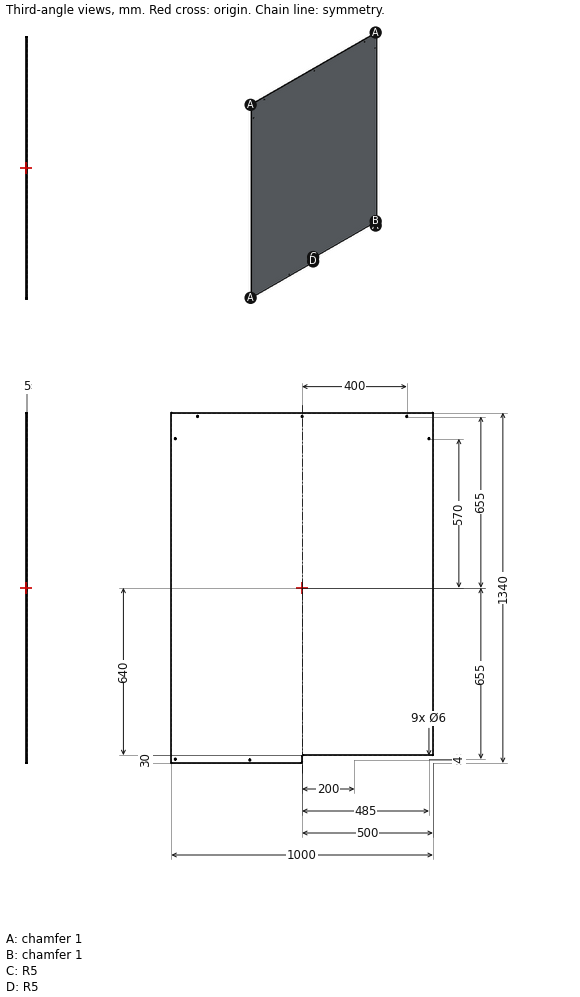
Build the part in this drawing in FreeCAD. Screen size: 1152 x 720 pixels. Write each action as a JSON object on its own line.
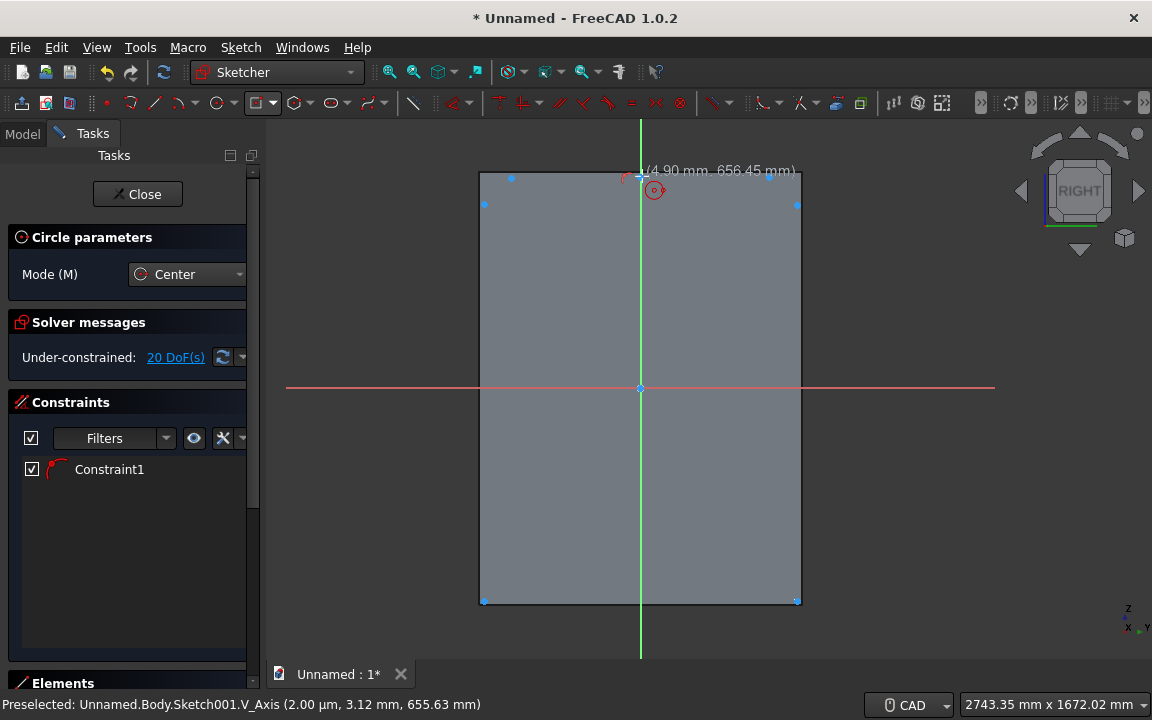
{"action": "scroll", "coordinate": [705, 601], "scroll_direction": "up", "scroll_amount": 16}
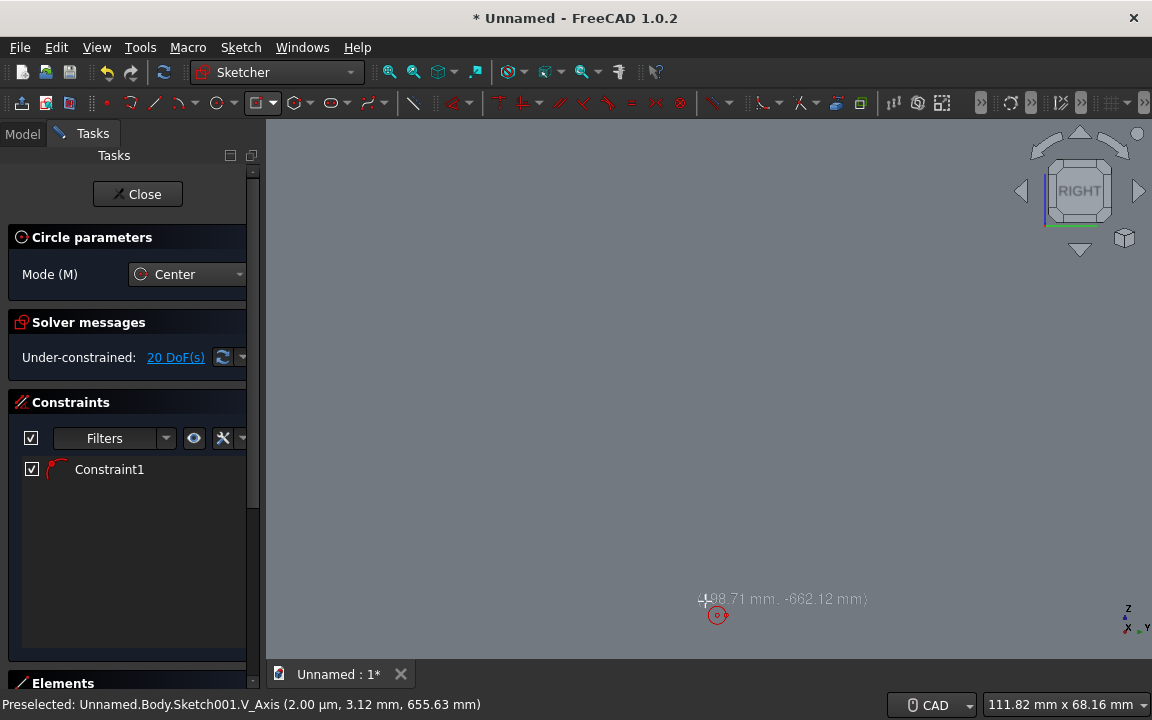
{"action": "scroll", "coordinate": [705, 602], "scroll_direction": "down", "scroll_amount": 16}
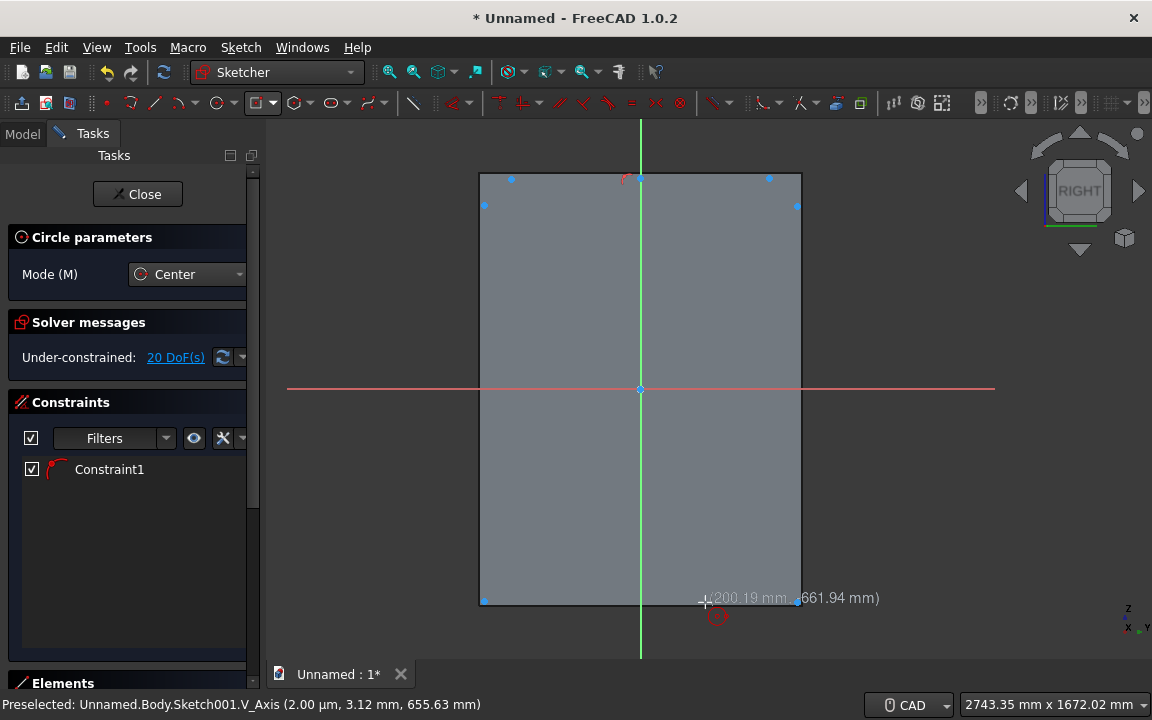
{"action": "left_click", "coordinate": [705, 602]}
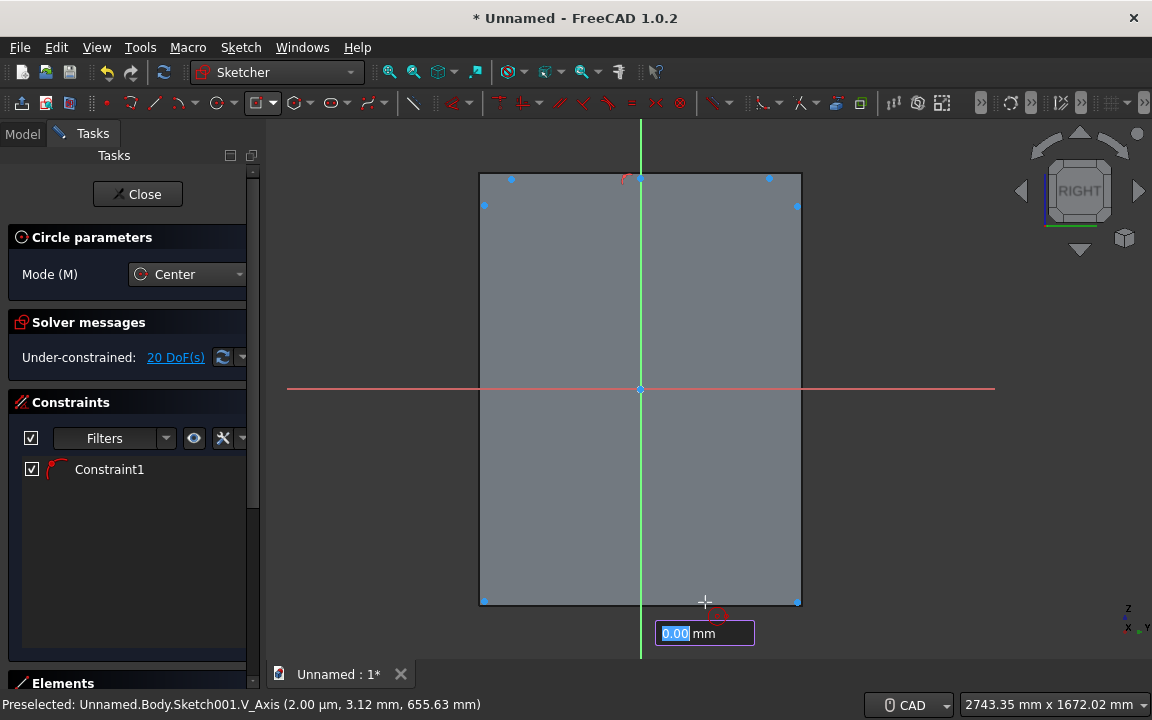
{"action": "scroll", "coordinate": [706, 601], "scroll_direction": "up", "scroll_amount": 14}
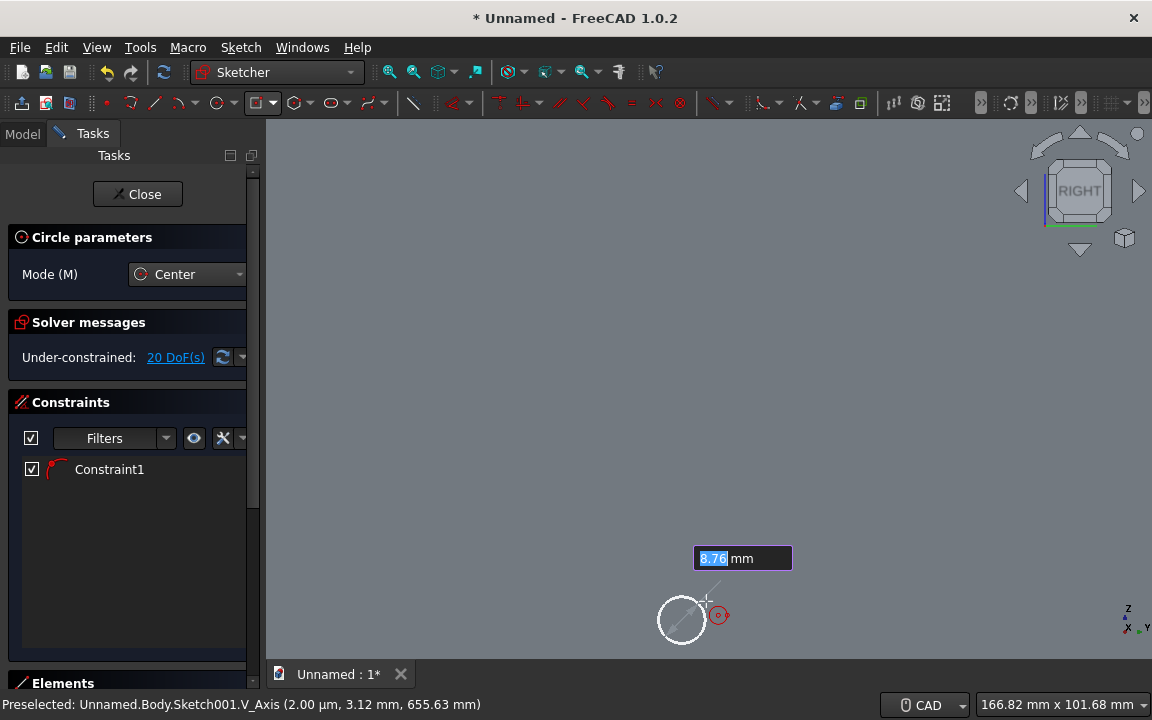
{"action": "left_click", "coordinate": [700, 592]}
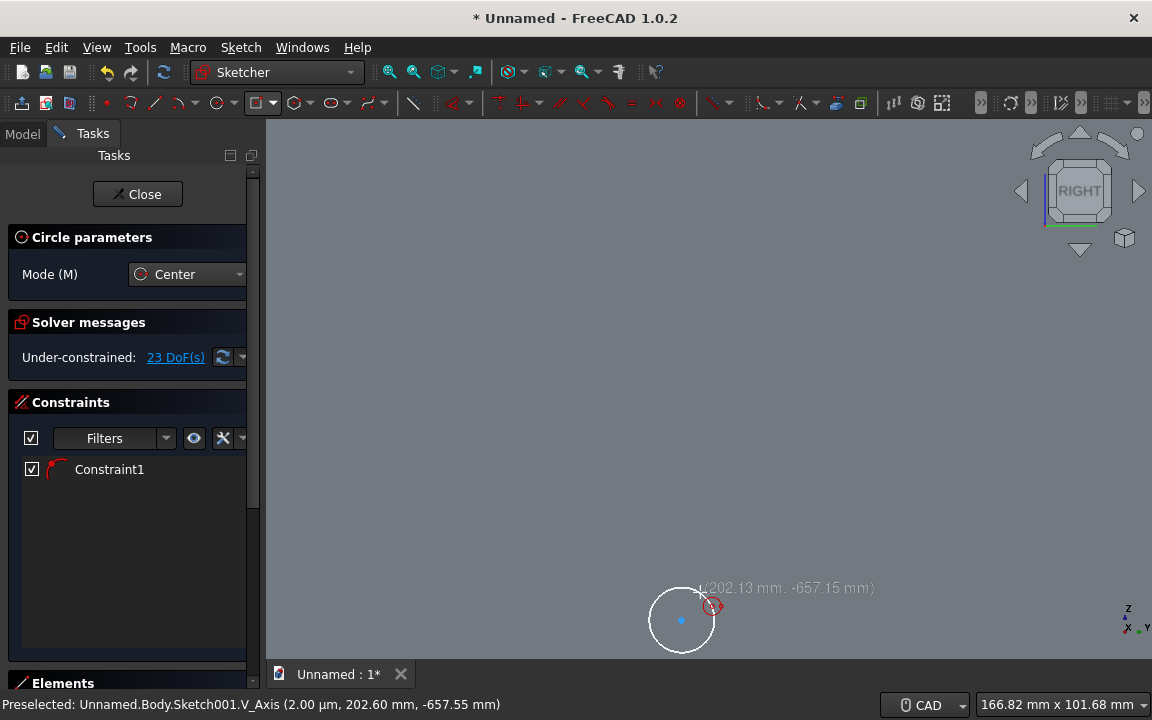
{"action": "scroll", "coordinate": [694, 561], "scroll_direction": "down", "scroll_amount": 15}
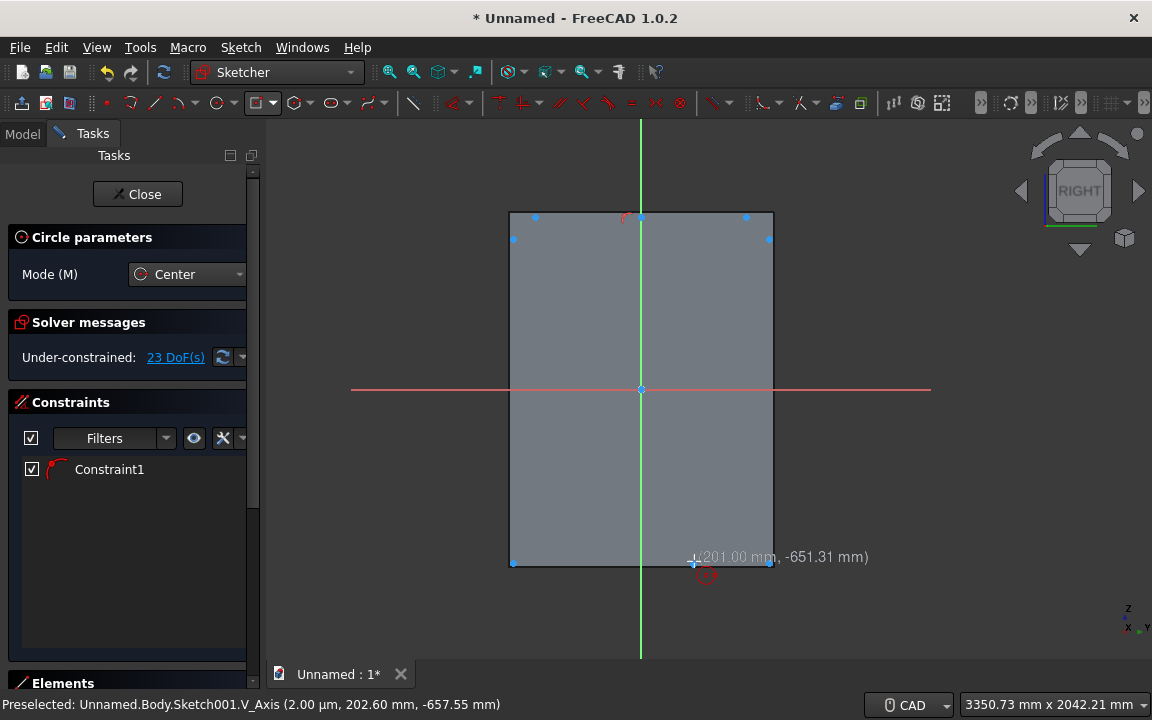
{"action": "scroll", "coordinate": [588, 564], "scroll_direction": "up", "scroll_amount": 17}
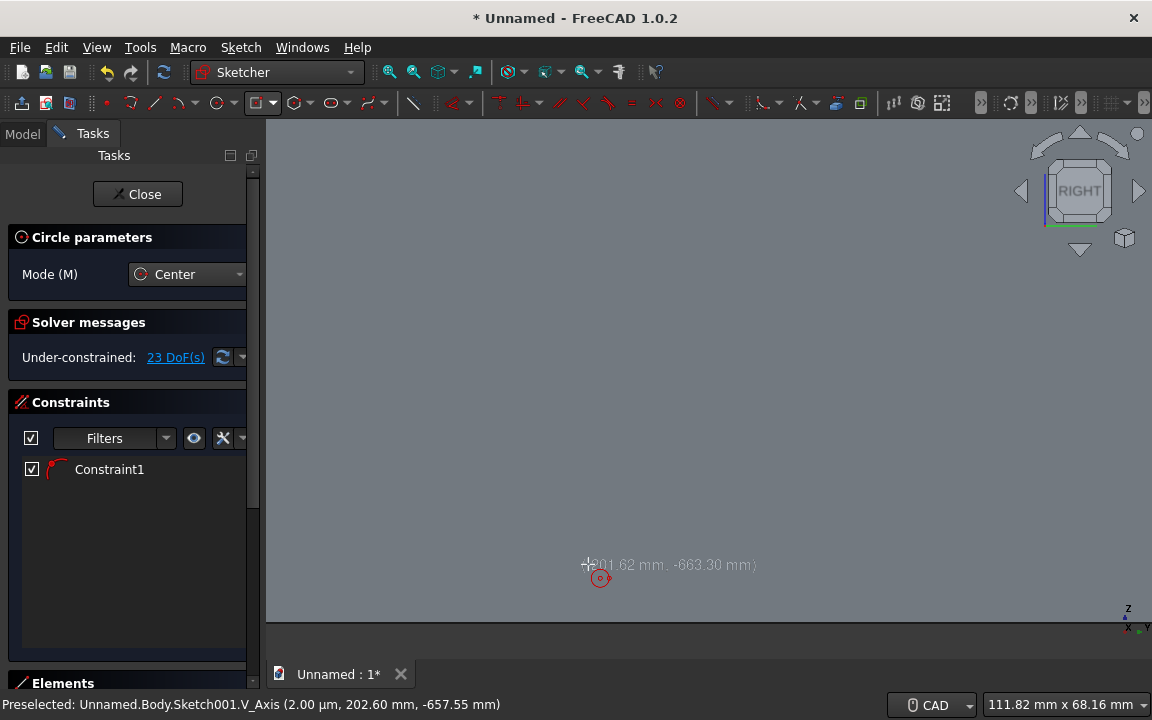
{"action": "scroll", "coordinate": [575, 604], "scroll_direction": "down", "scroll_amount": 16}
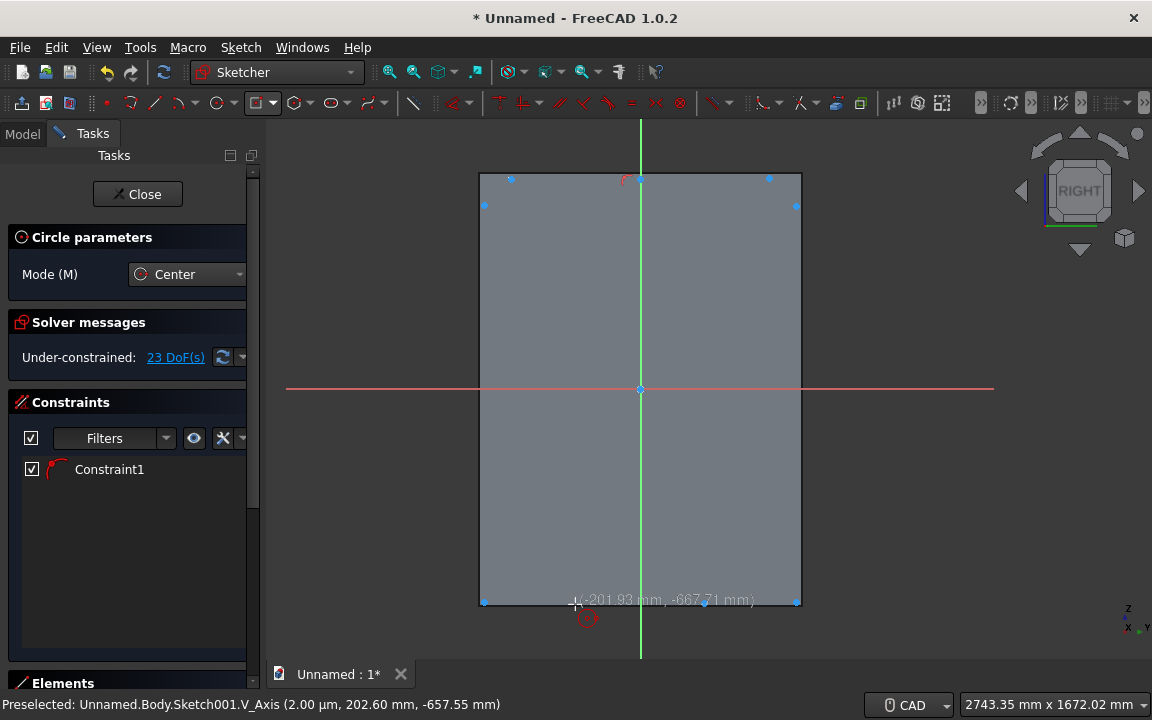
{"action": "left_click", "coordinate": [576, 602]}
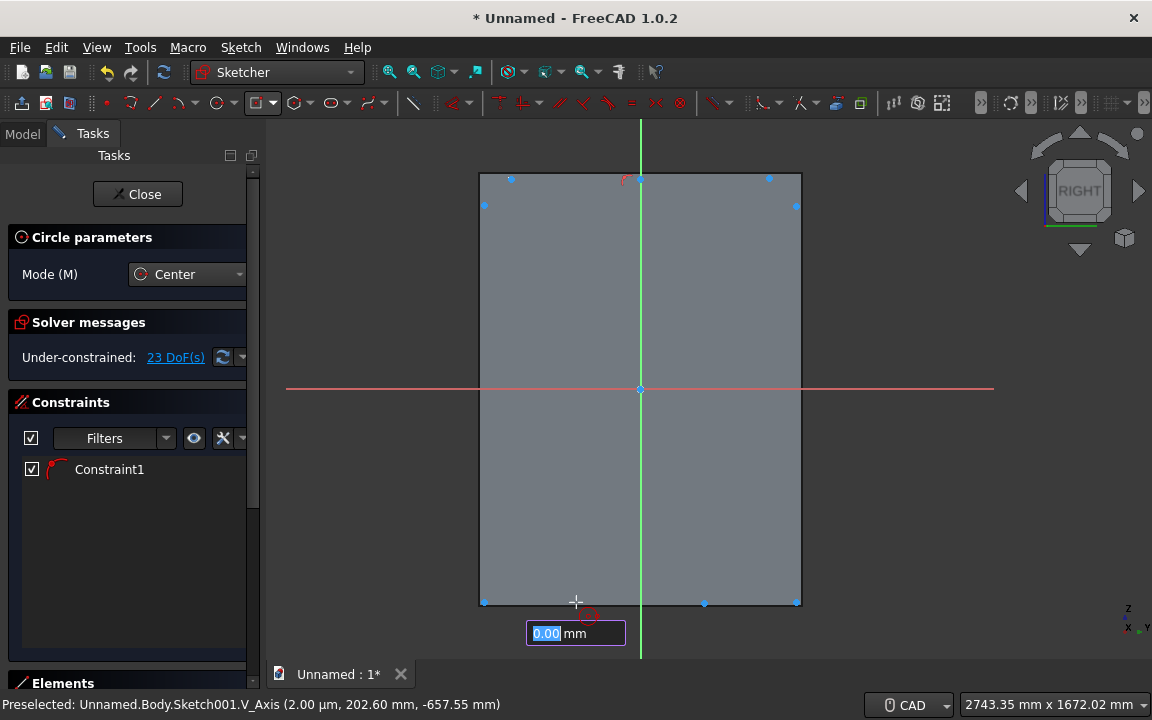
{"action": "scroll", "coordinate": [577, 601], "scroll_direction": "up", "scroll_amount": 14}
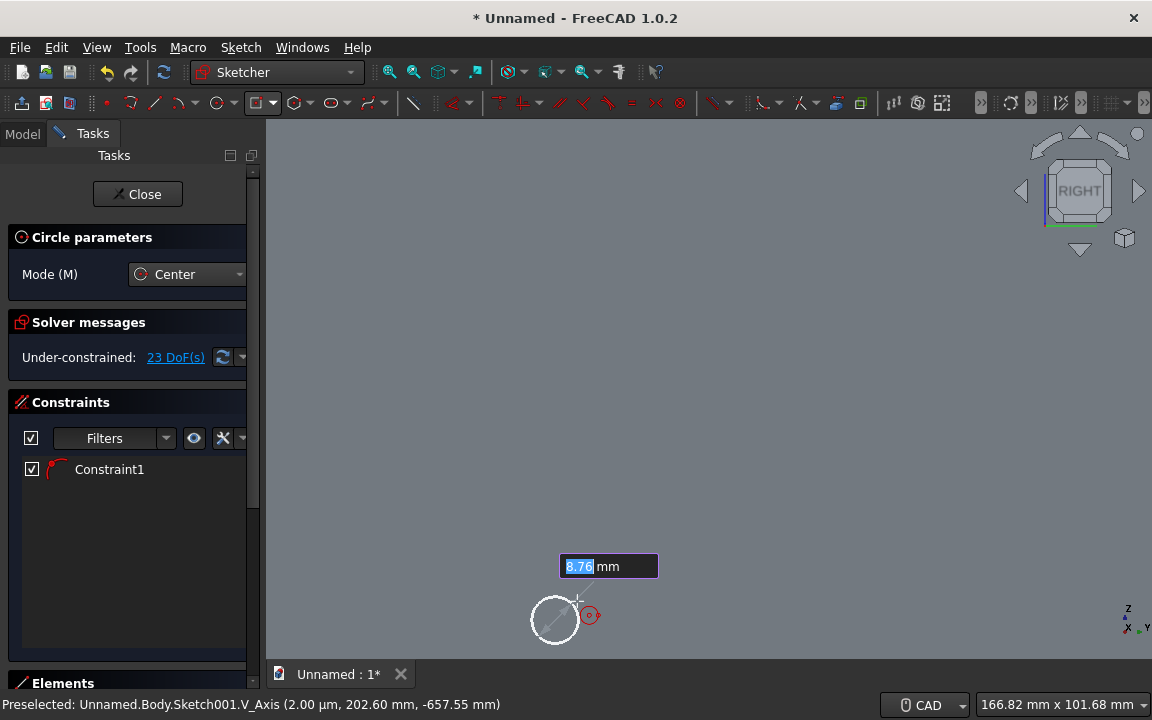
{"action": "left_click", "coordinate": [566, 594]}
{"action": "key", "text": "Escape"}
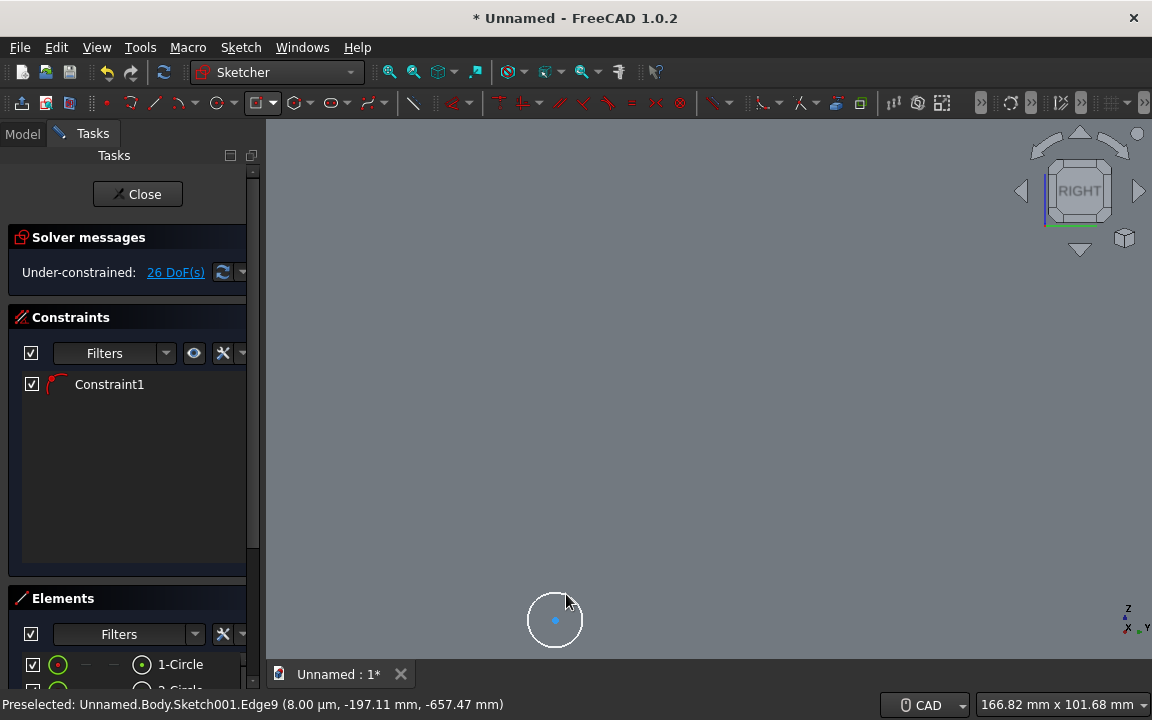
{"action": "scroll", "coordinate": [589, 561], "scroll_direction": "down", "scroll_amount": 15}